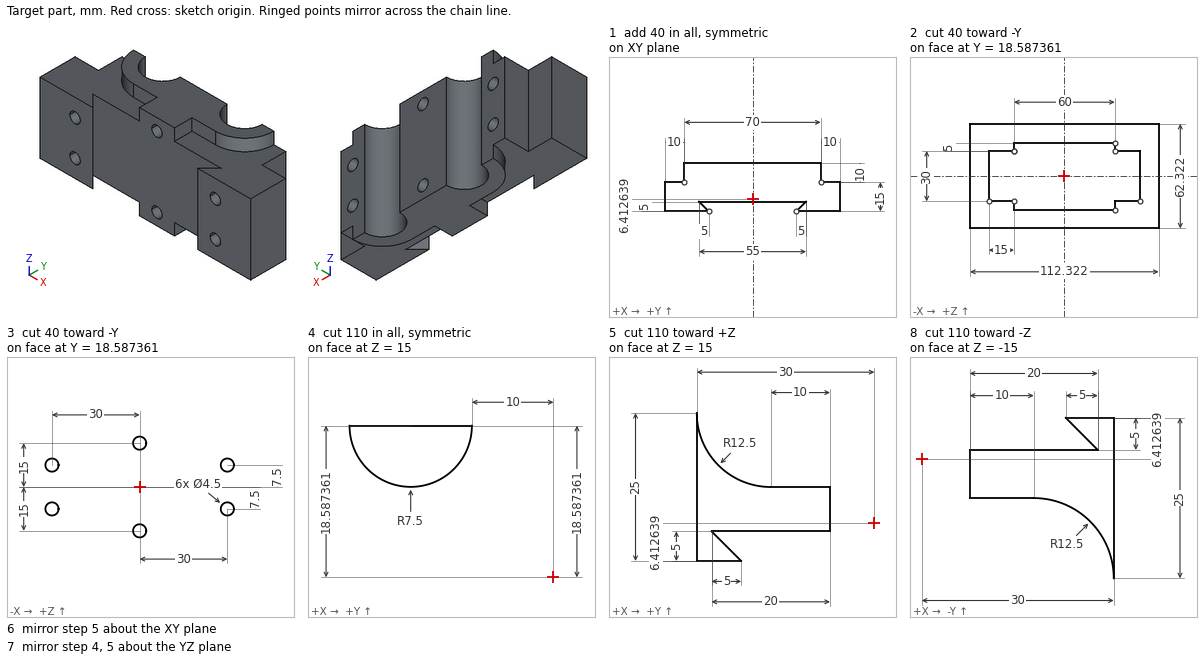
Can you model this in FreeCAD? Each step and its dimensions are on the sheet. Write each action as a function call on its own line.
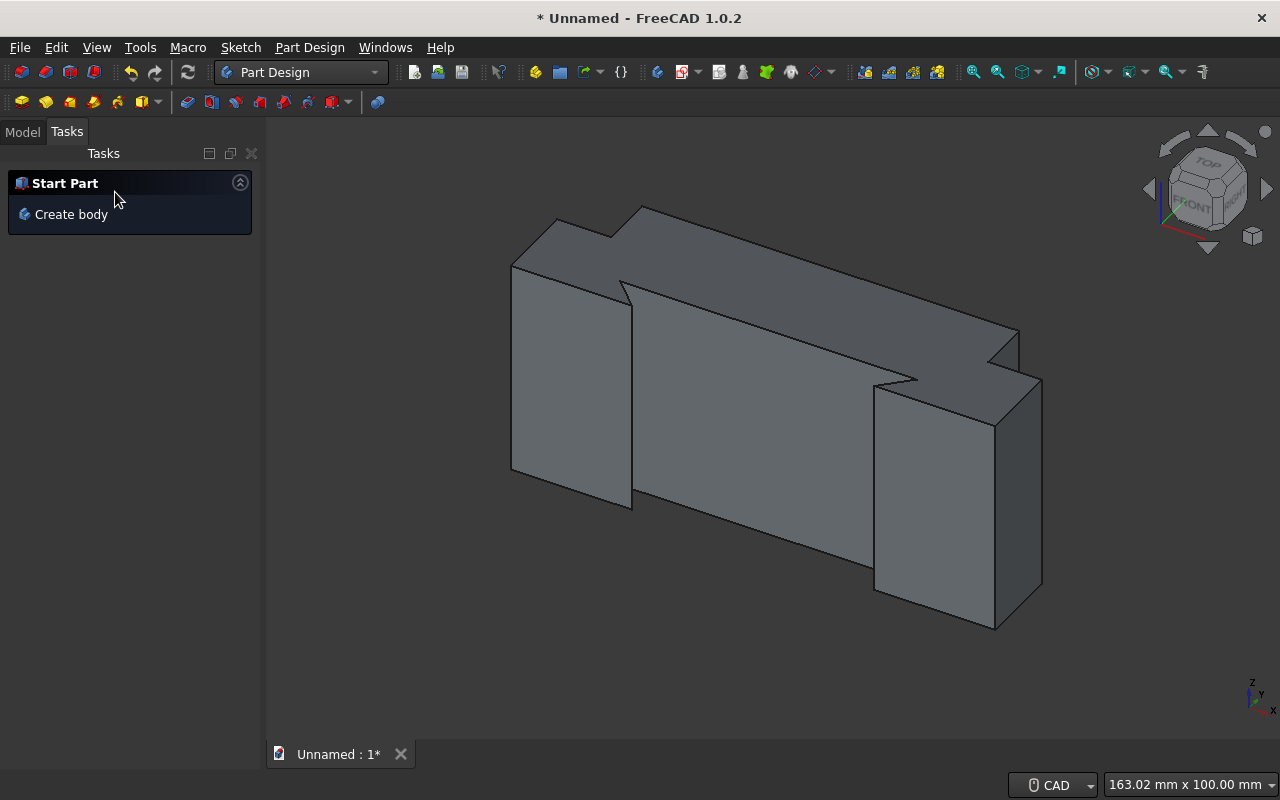
key(4)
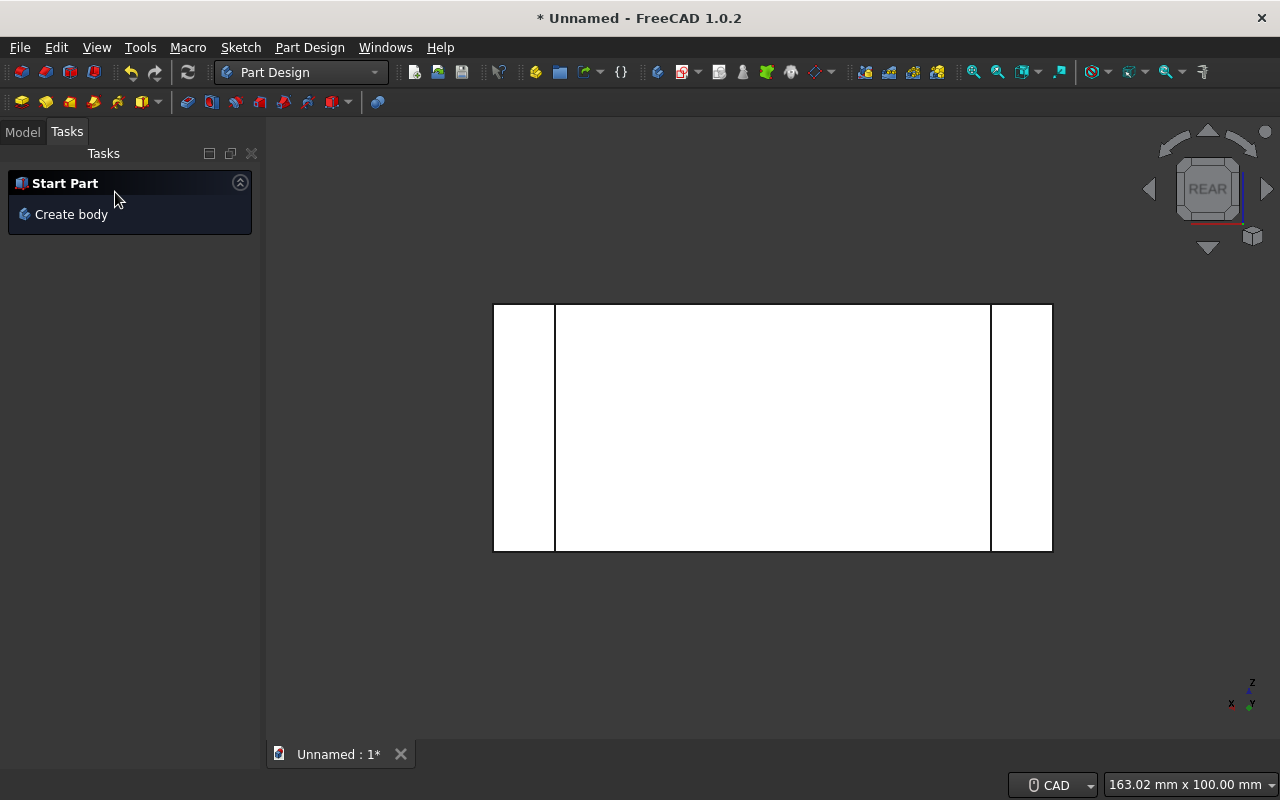
click(711, 427)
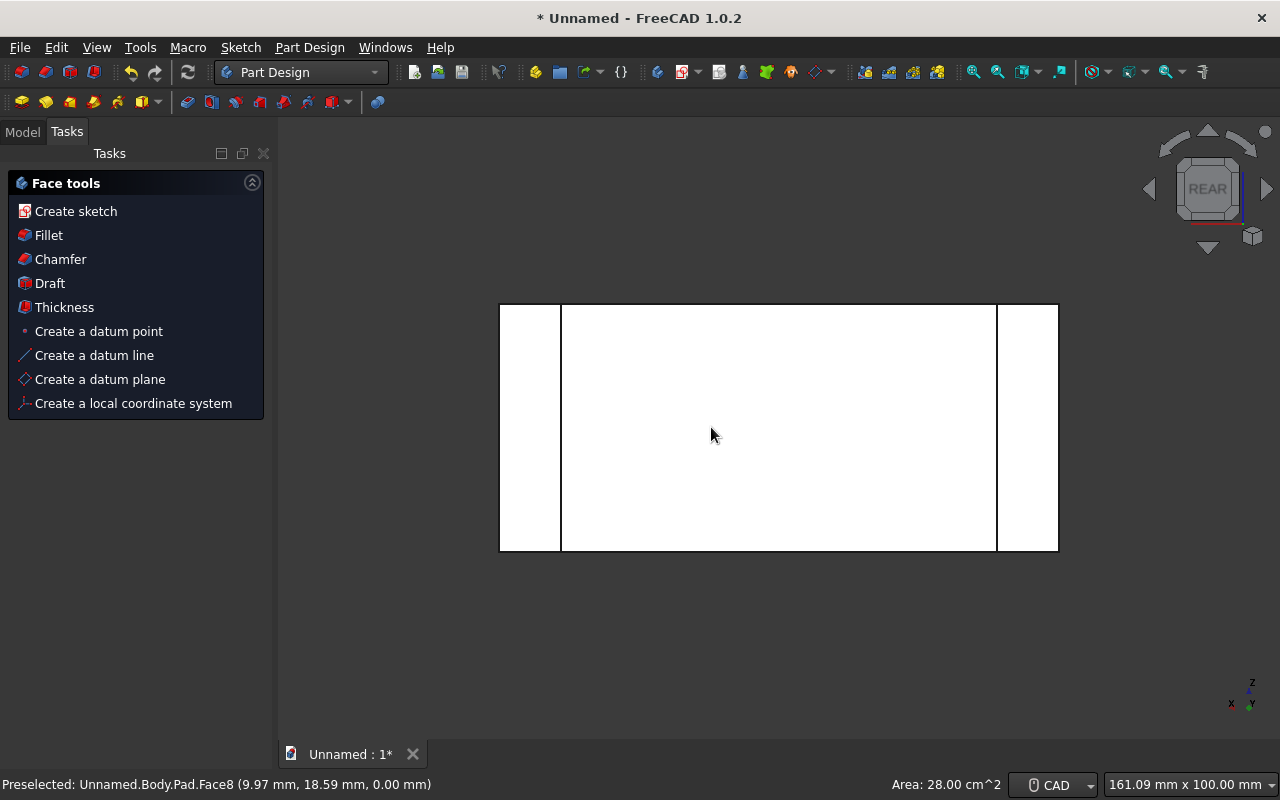
click(682, 72)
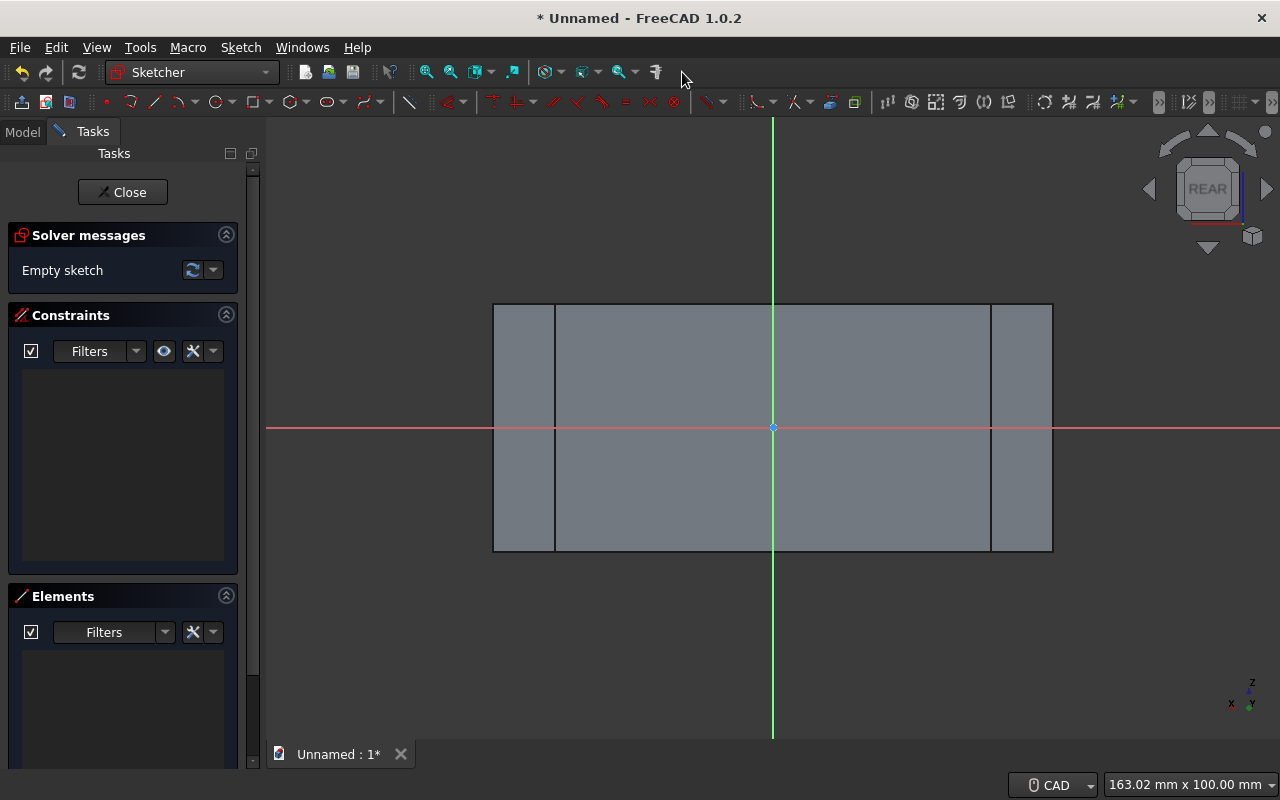
scroll(395, 428, down, 1)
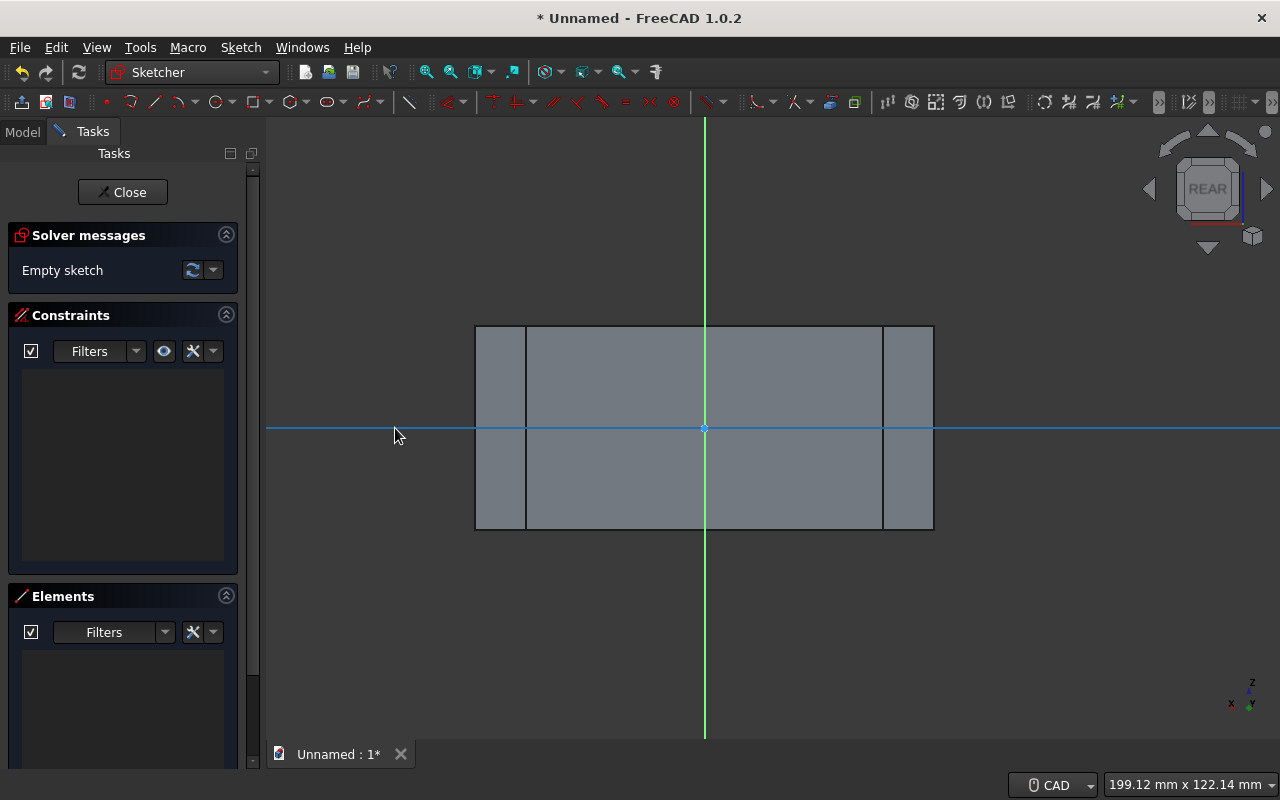
click(272, 102)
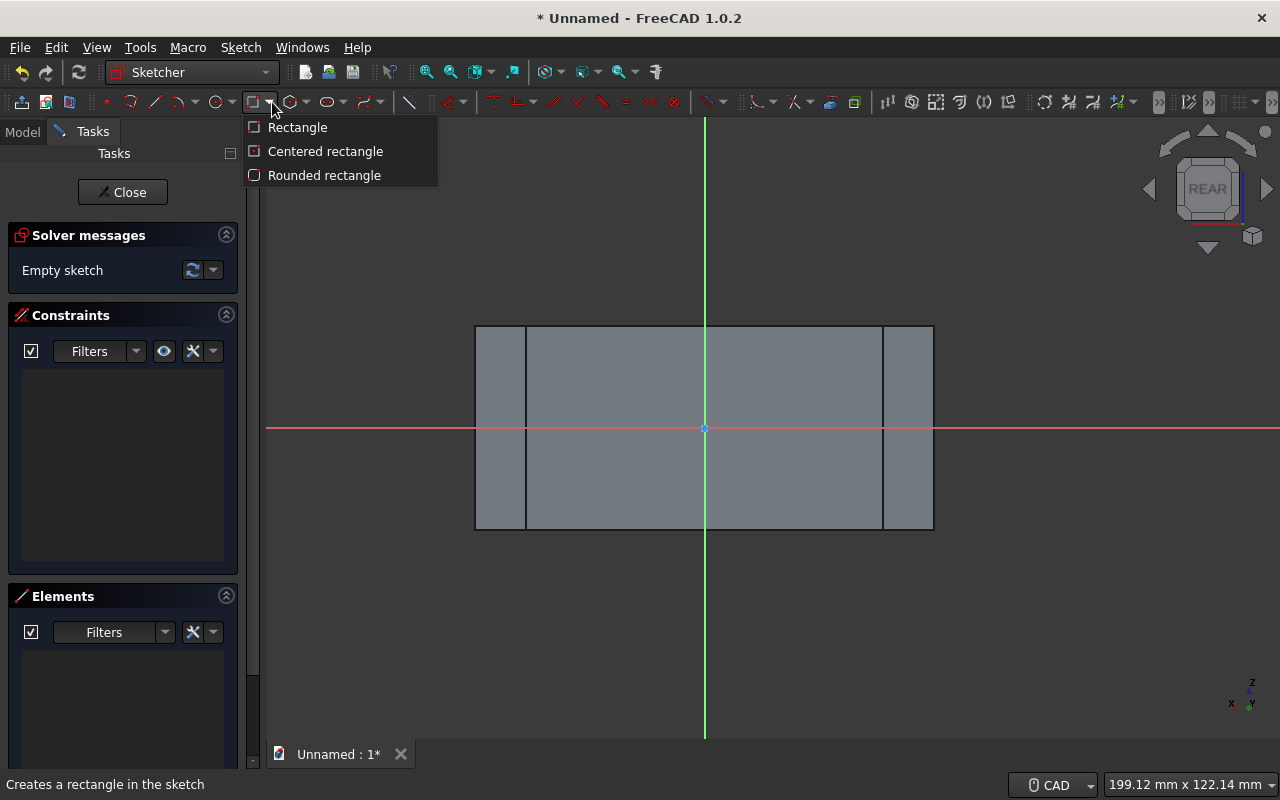
click(340, 151)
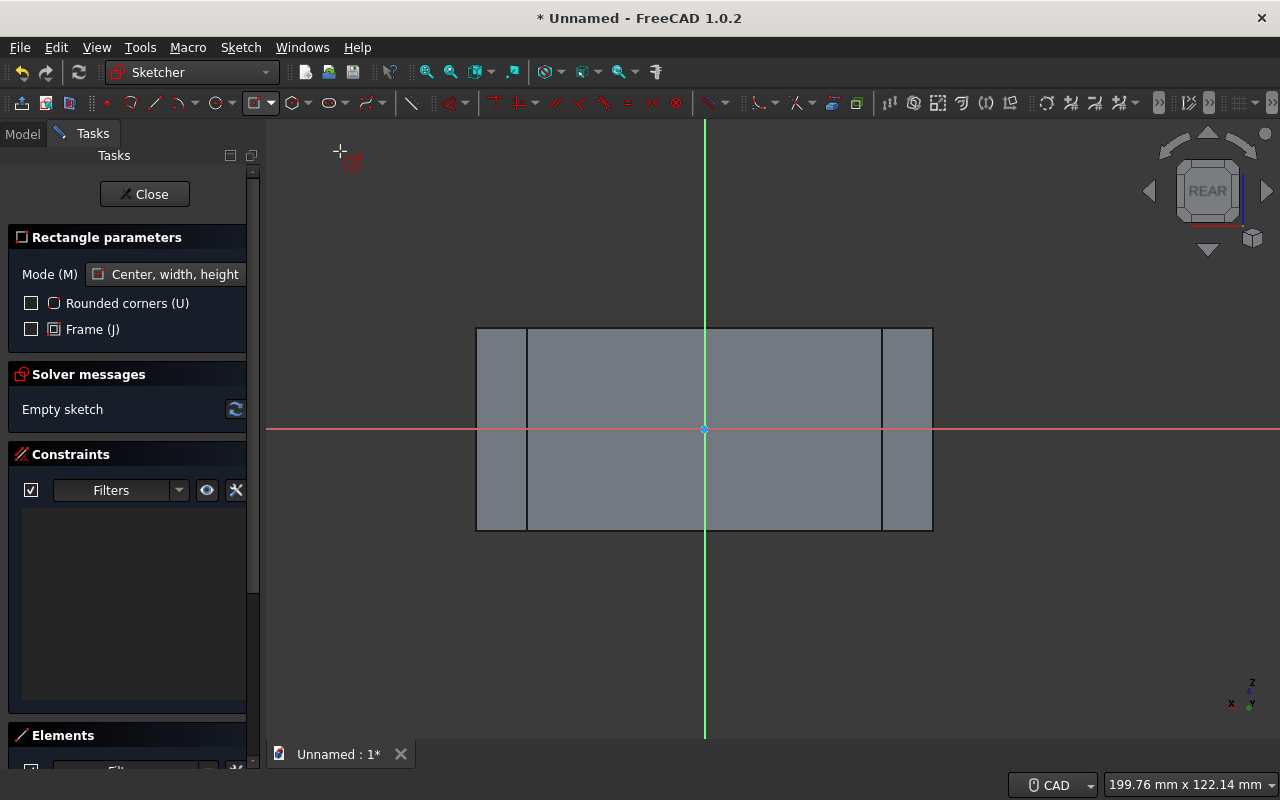
click(705, 429)
click(990, 271)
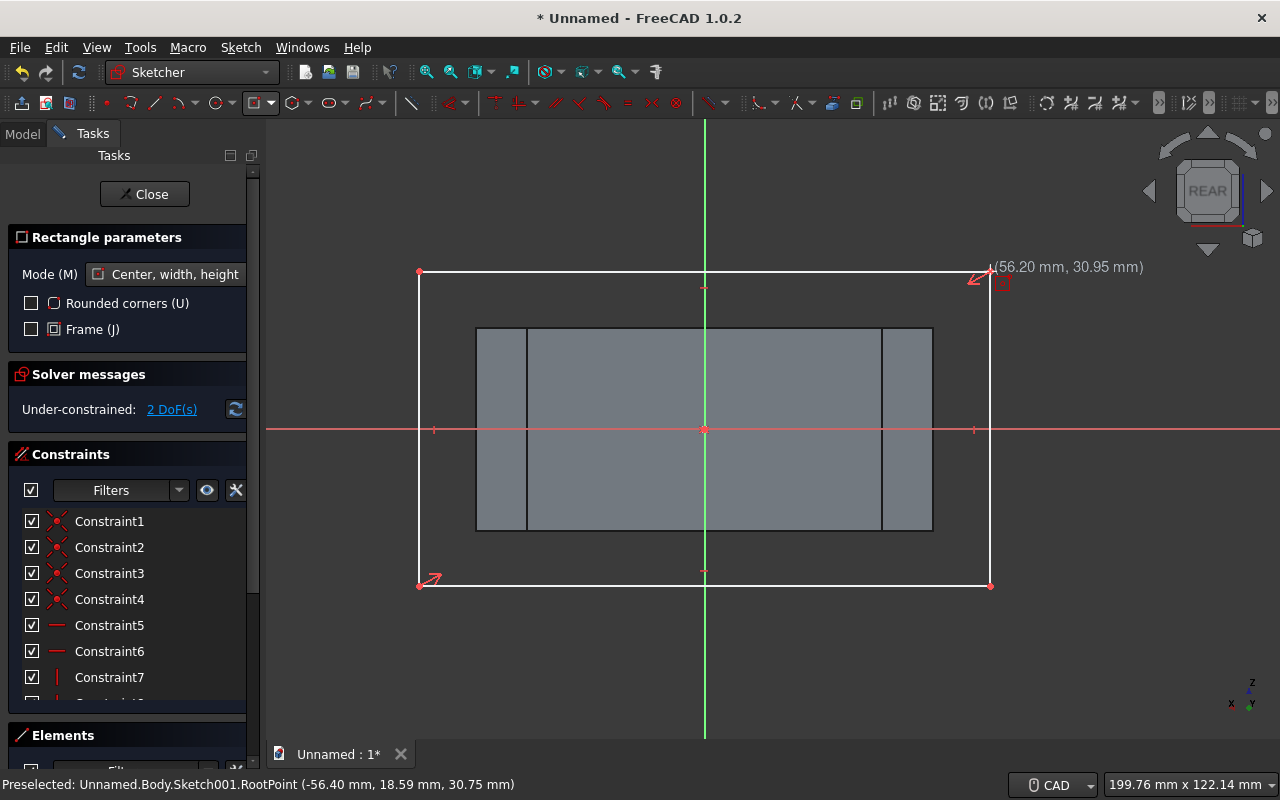
click(132, 104)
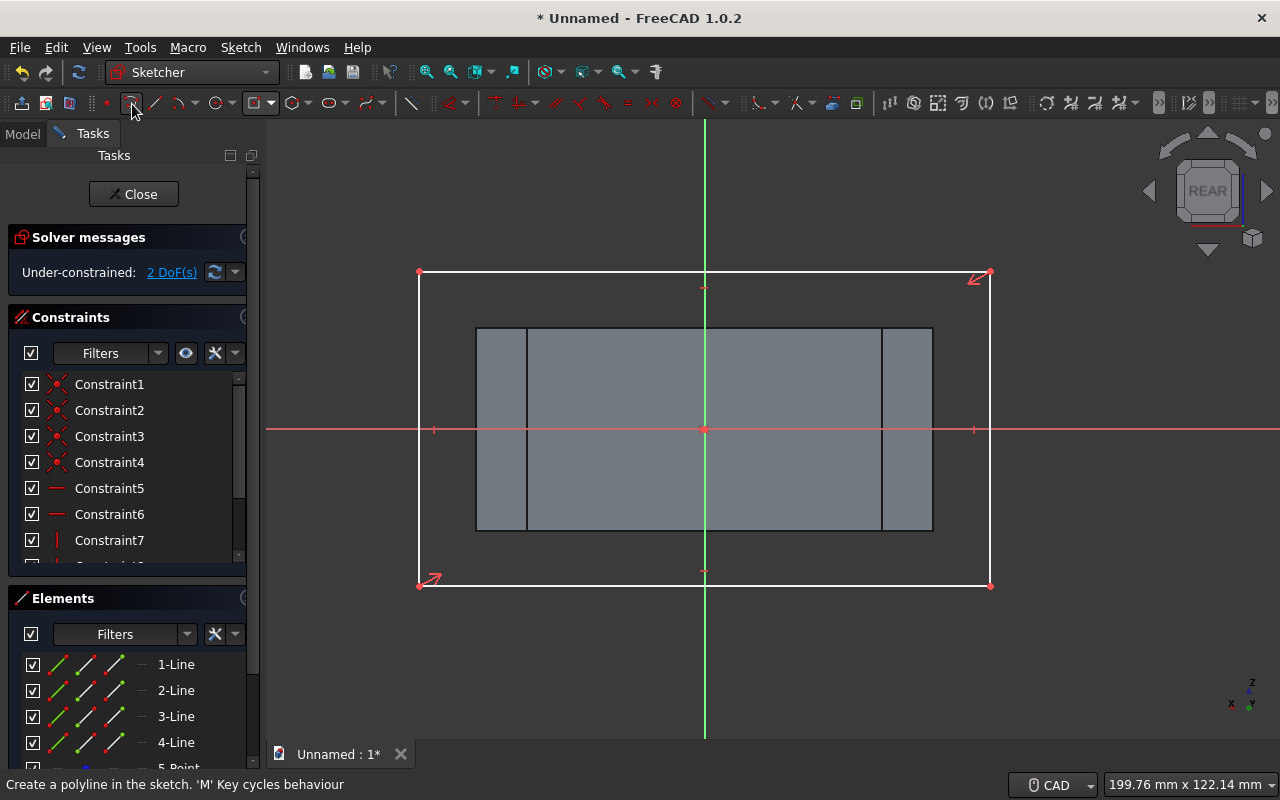
click(552, 505)
click(476, 505)
click(476, 353)
click(552, 353)
click(552, 328)
click(857, 328)
click(857, 353)
click(933, 353)
click(933, 505)
click(857, 505)
click(857, 531)
click(552, 531)
click(552, 506)
key(Escape)
key(Escape)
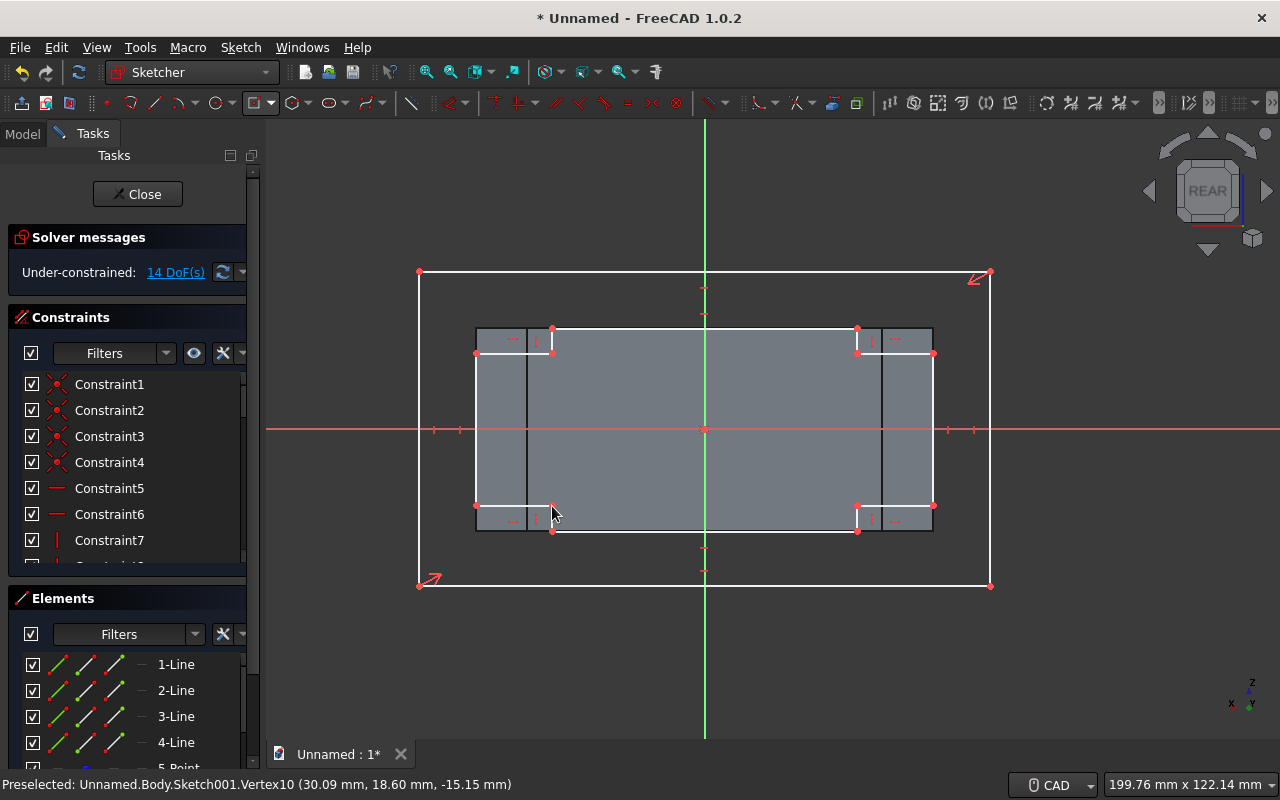
click(552, 506)